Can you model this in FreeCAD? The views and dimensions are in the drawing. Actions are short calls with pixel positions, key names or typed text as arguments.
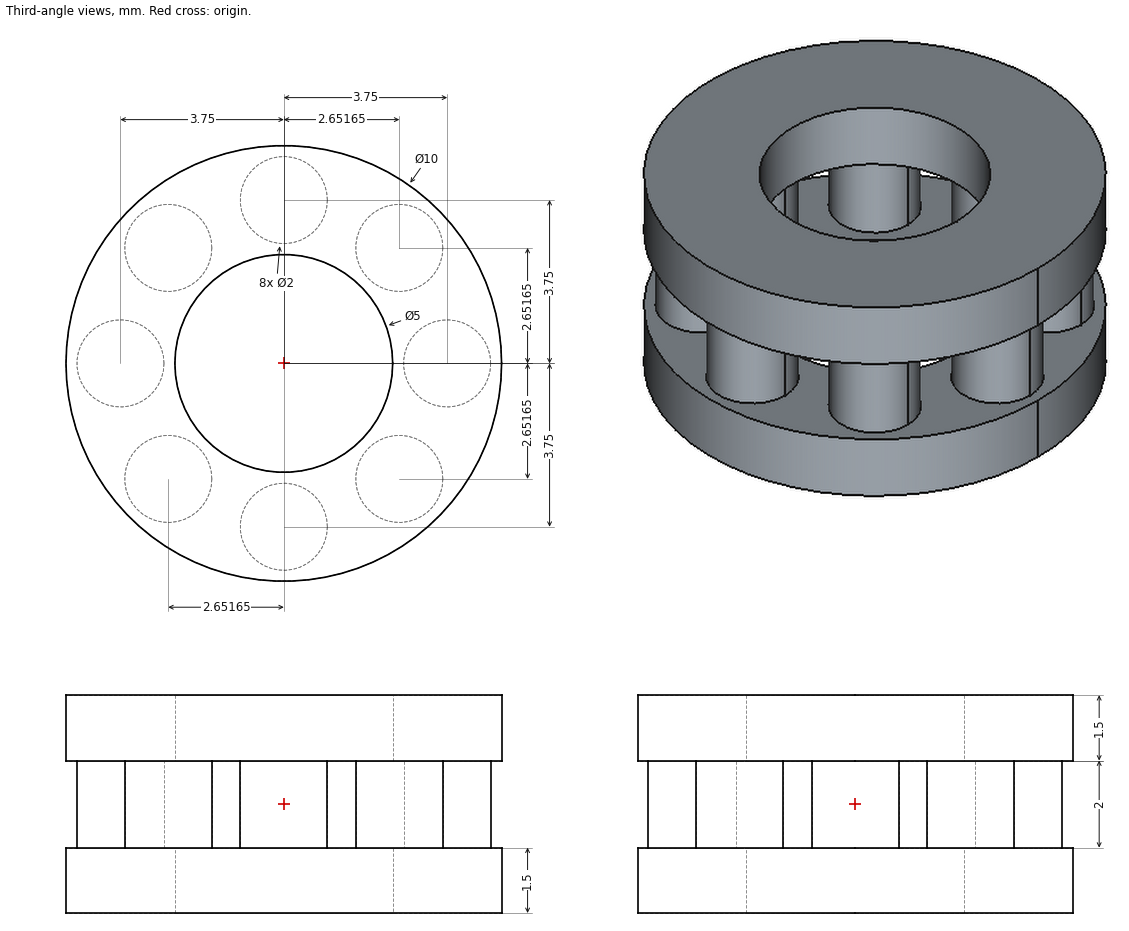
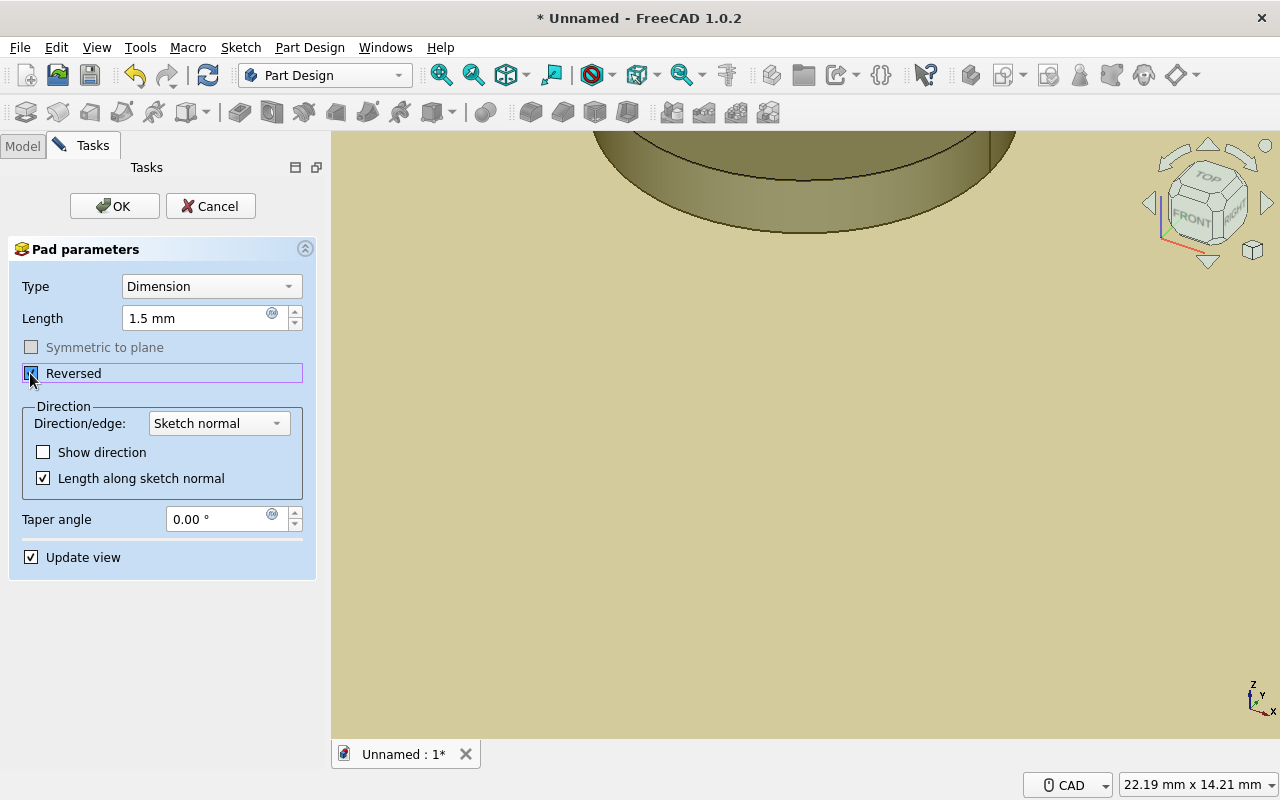
click(115, 206)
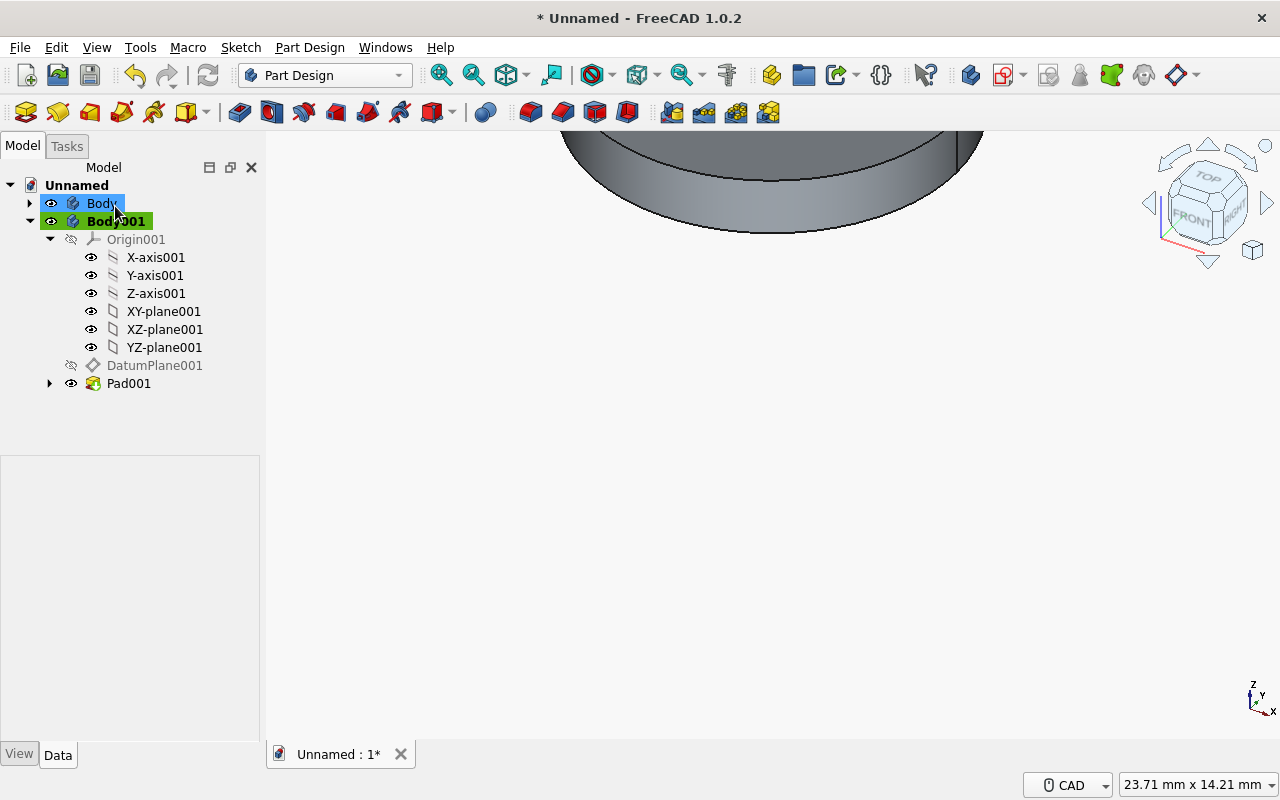
click(442, 76)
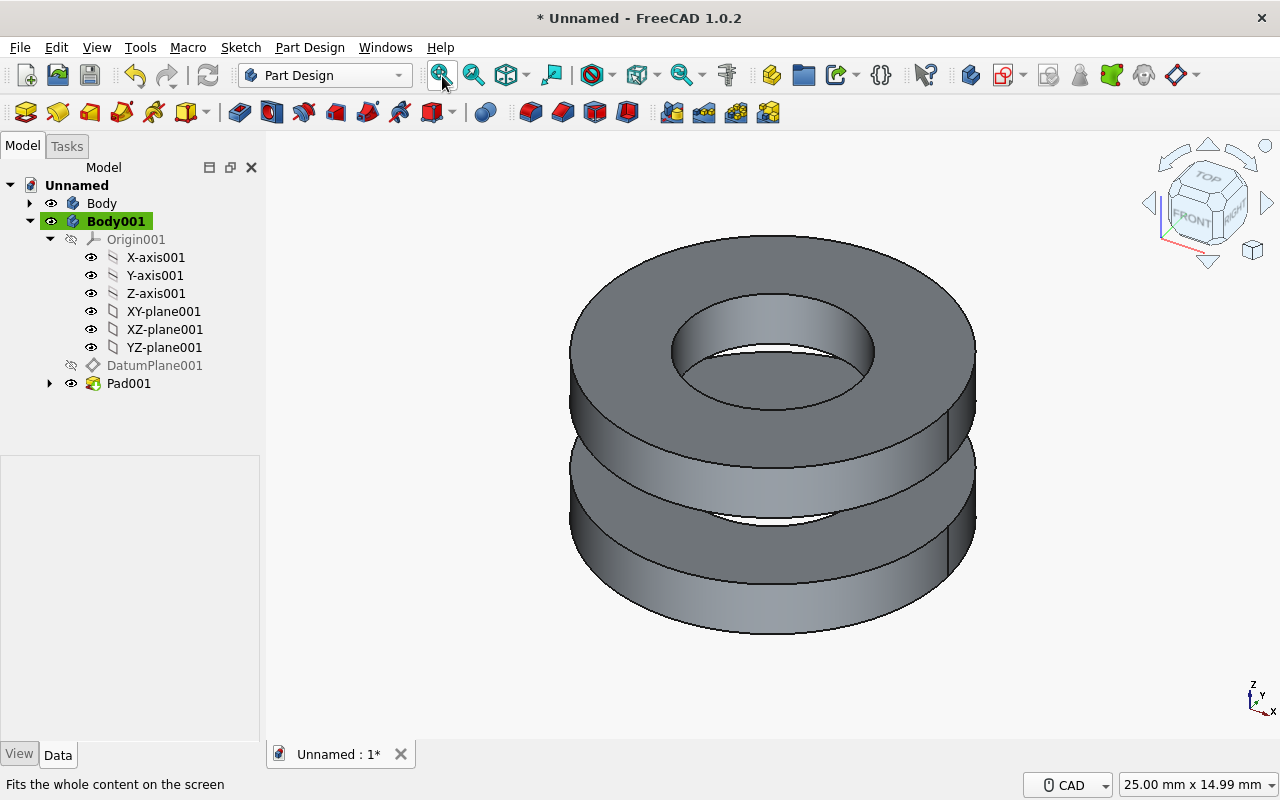
double_click(96, 203)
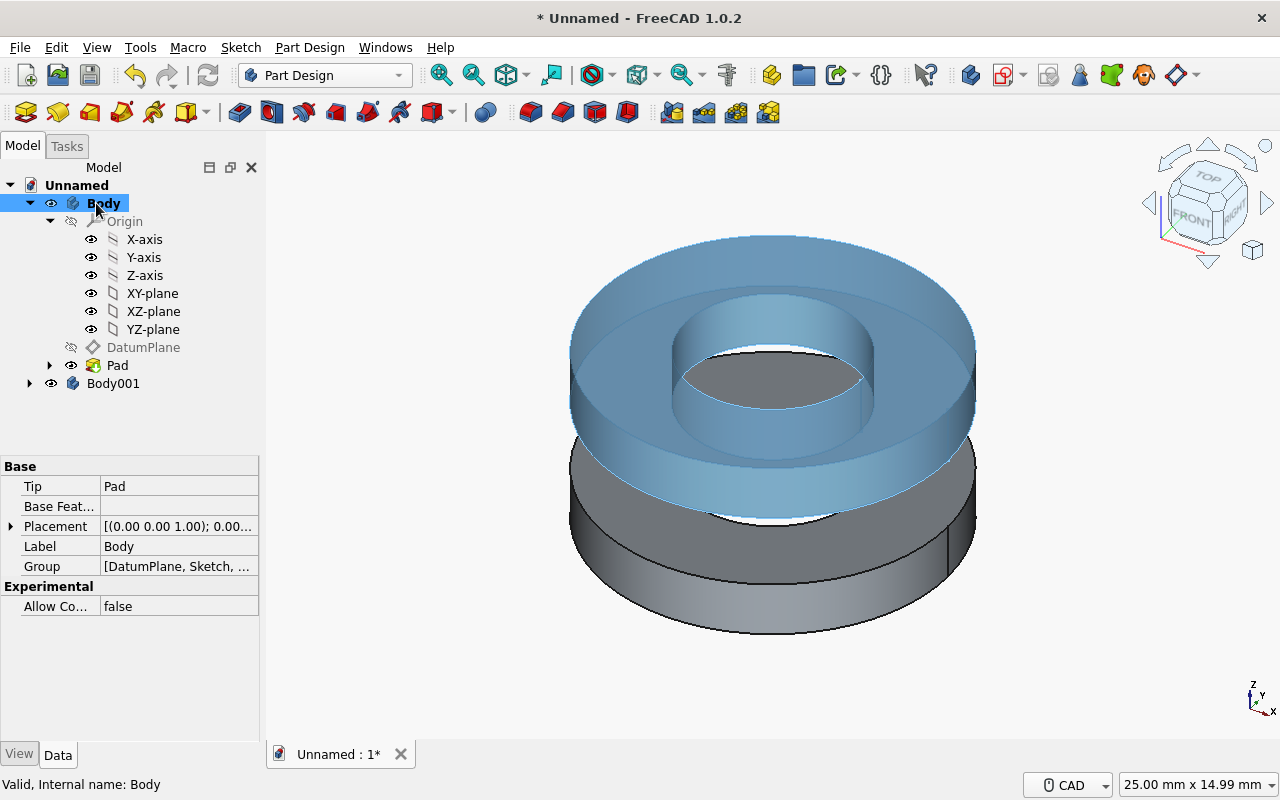
click(96, 203)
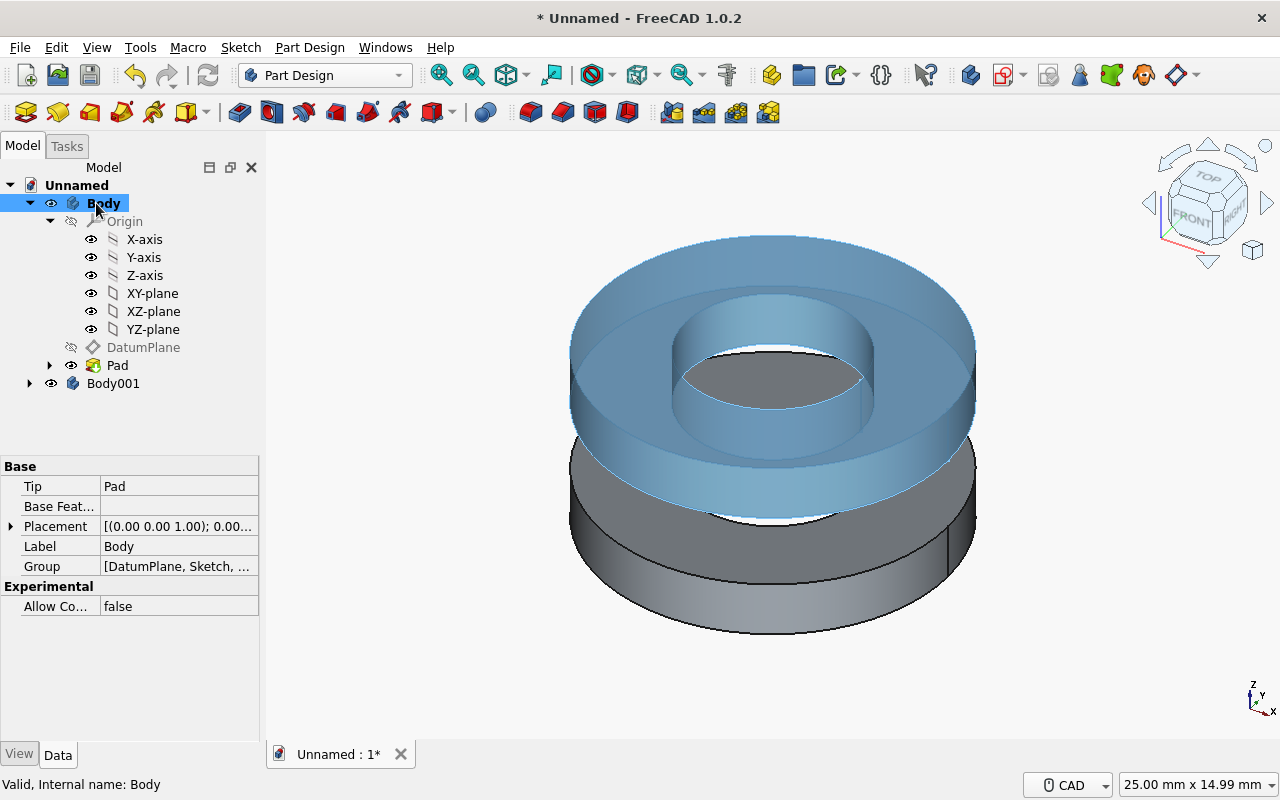
click(146, 606)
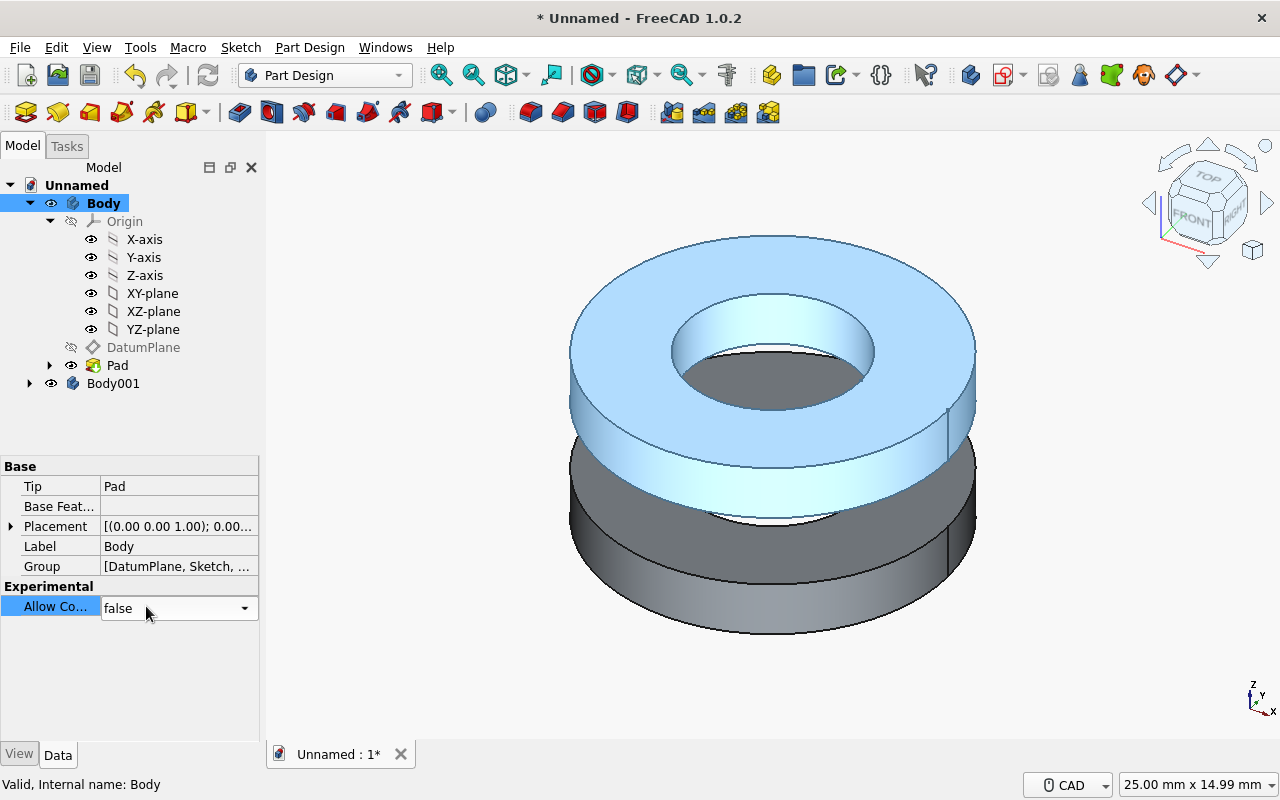
click(146, 606)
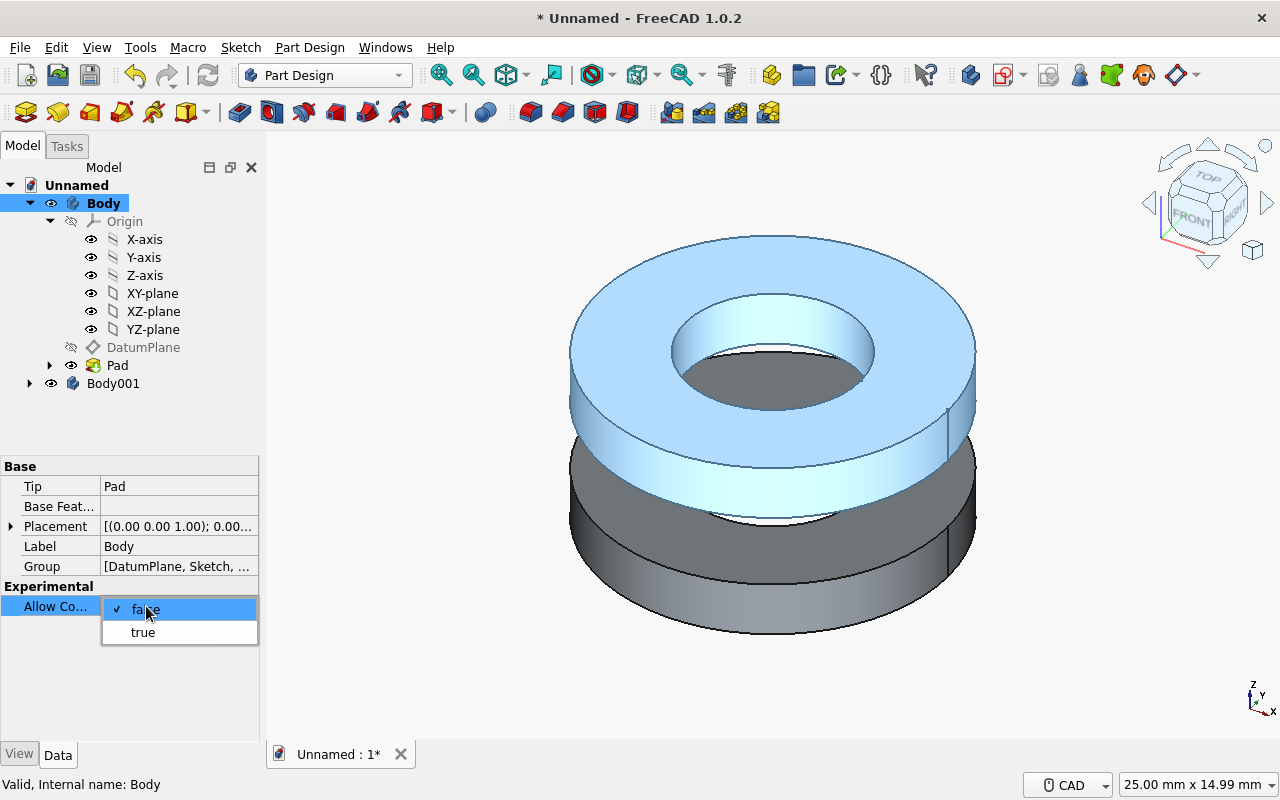
click(179, 632)
key(Return)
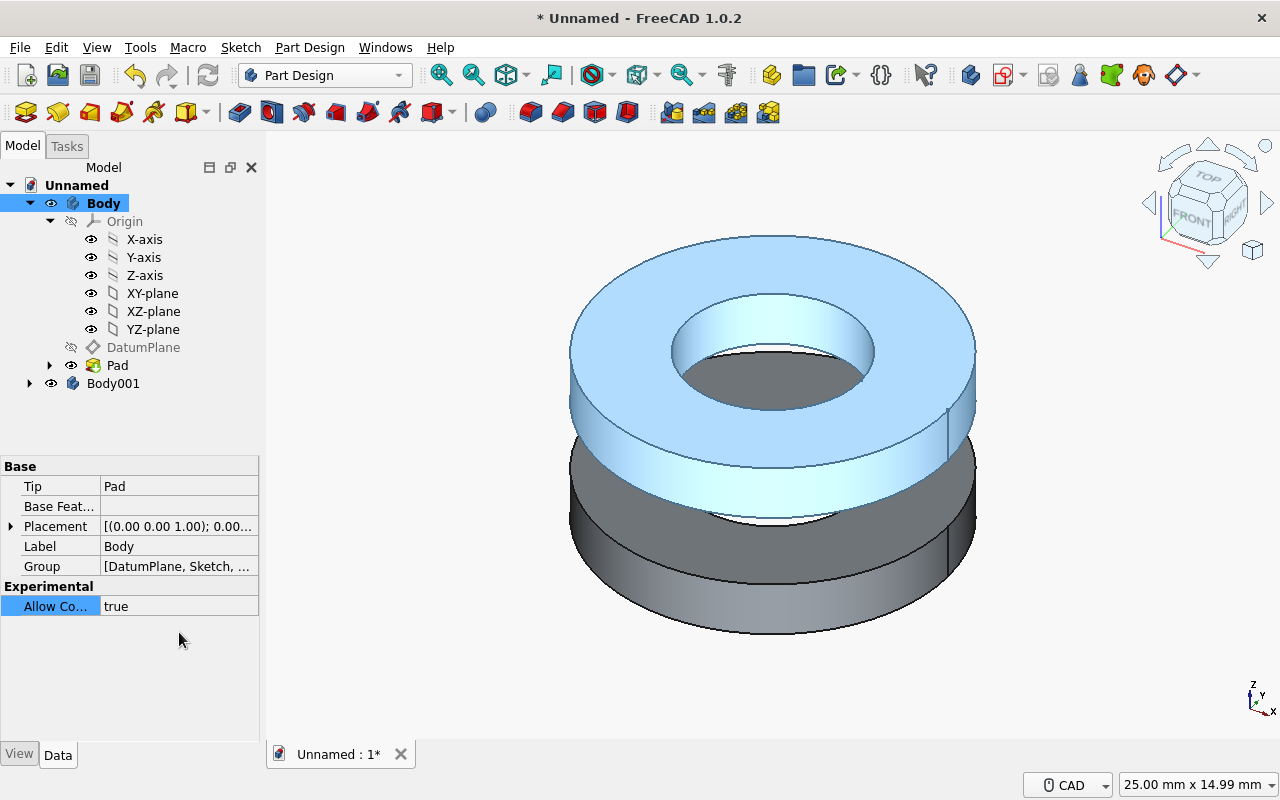
click(96, 383)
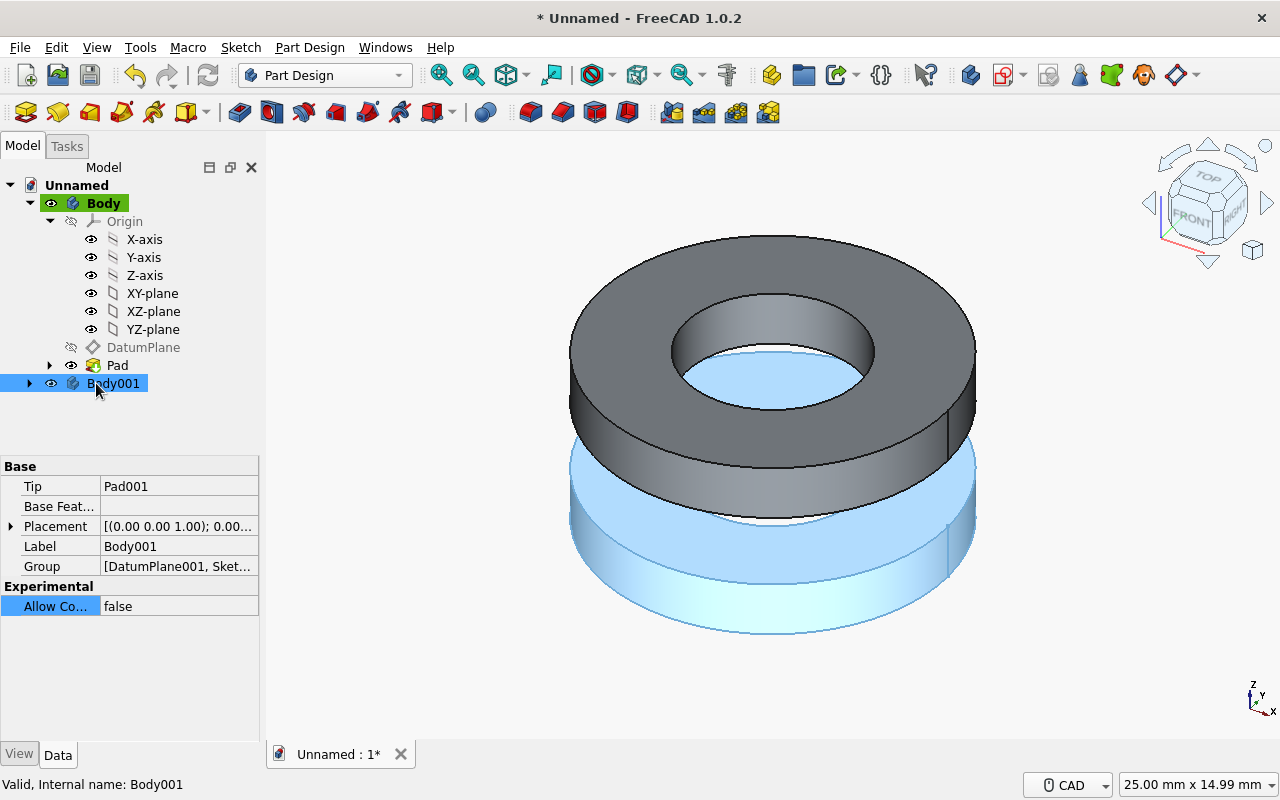
click(486, 112)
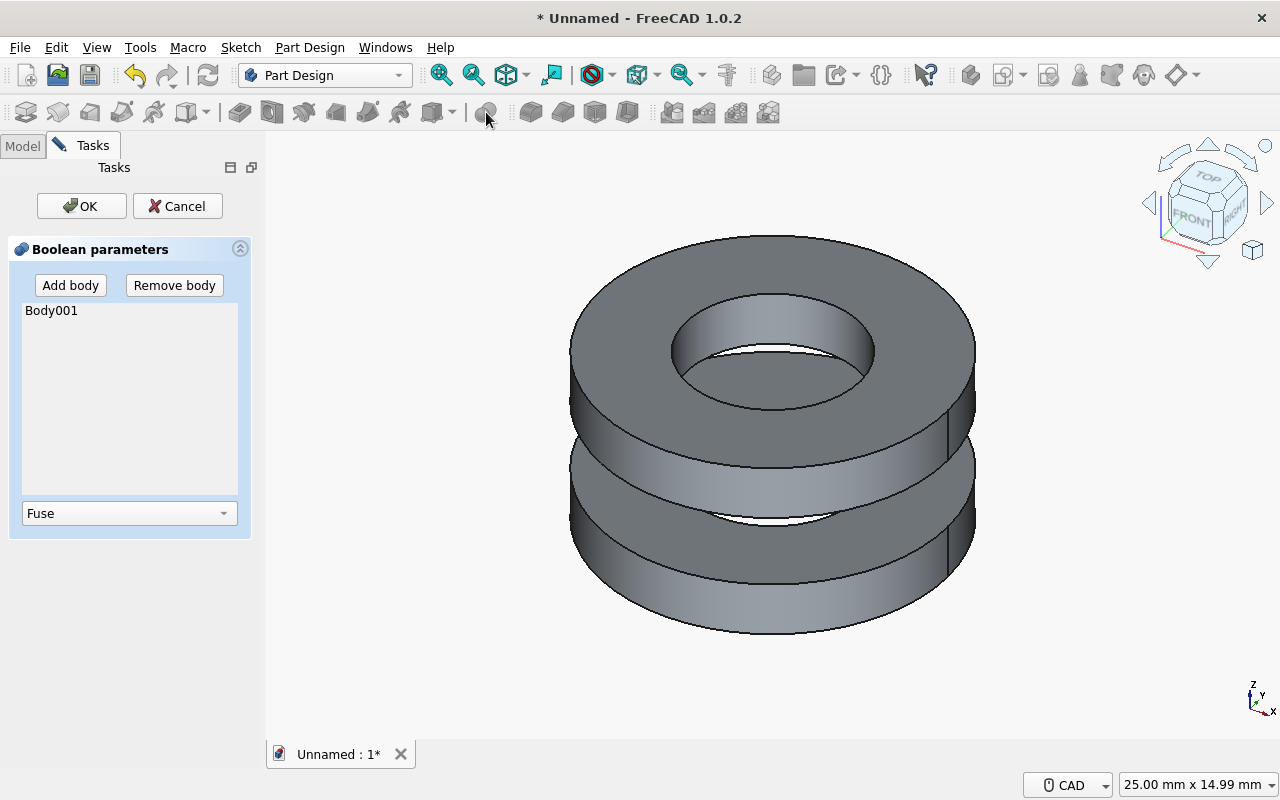
click(82, 206)